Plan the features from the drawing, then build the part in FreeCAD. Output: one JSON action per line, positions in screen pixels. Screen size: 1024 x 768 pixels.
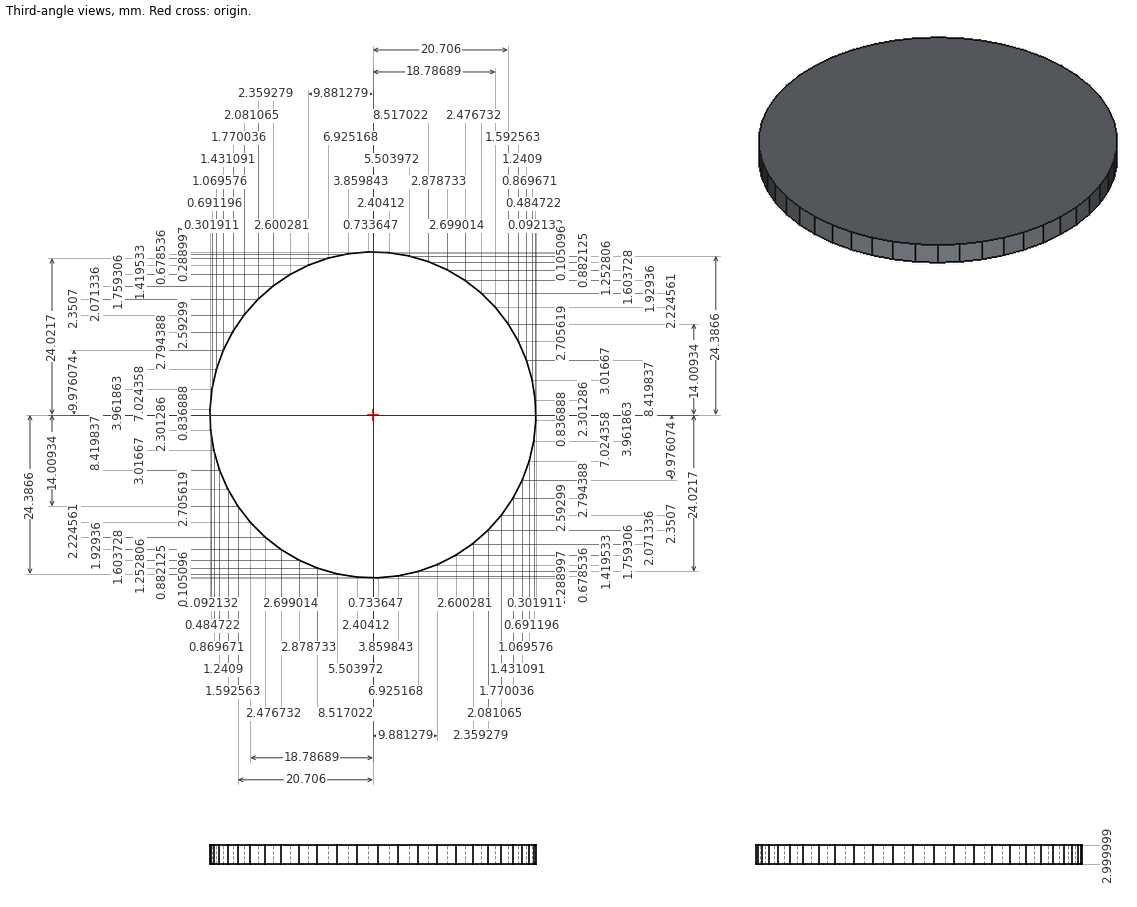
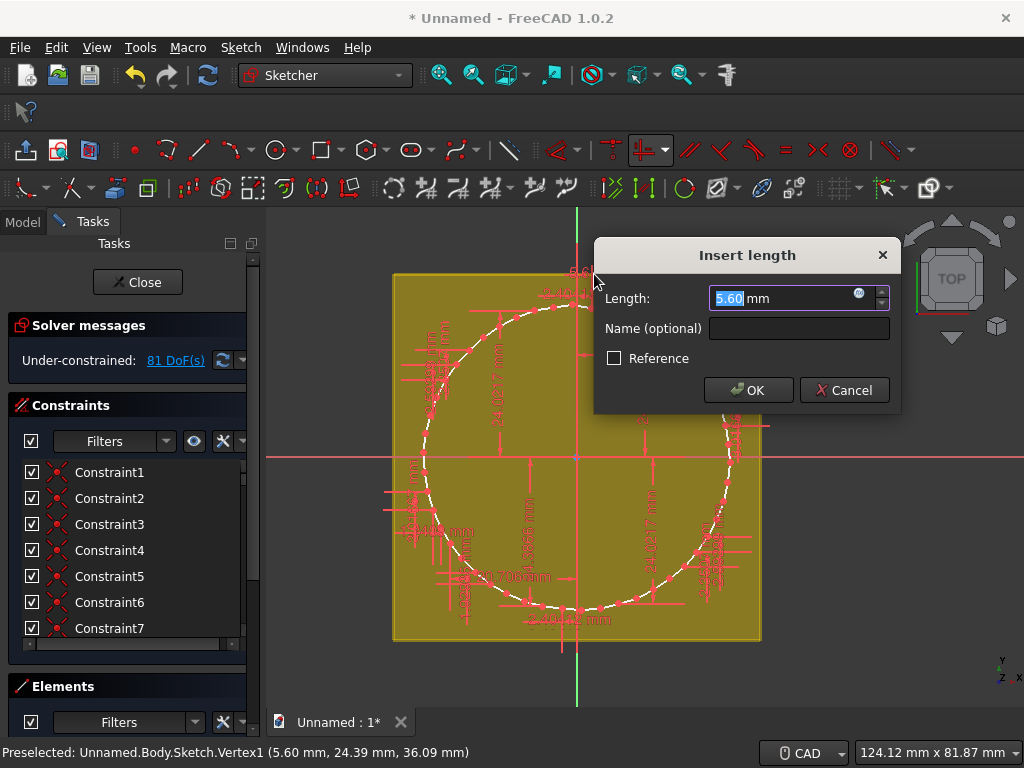
{"action": "type", "text": "5.503972"}
{"action": "key", "text": "Return"}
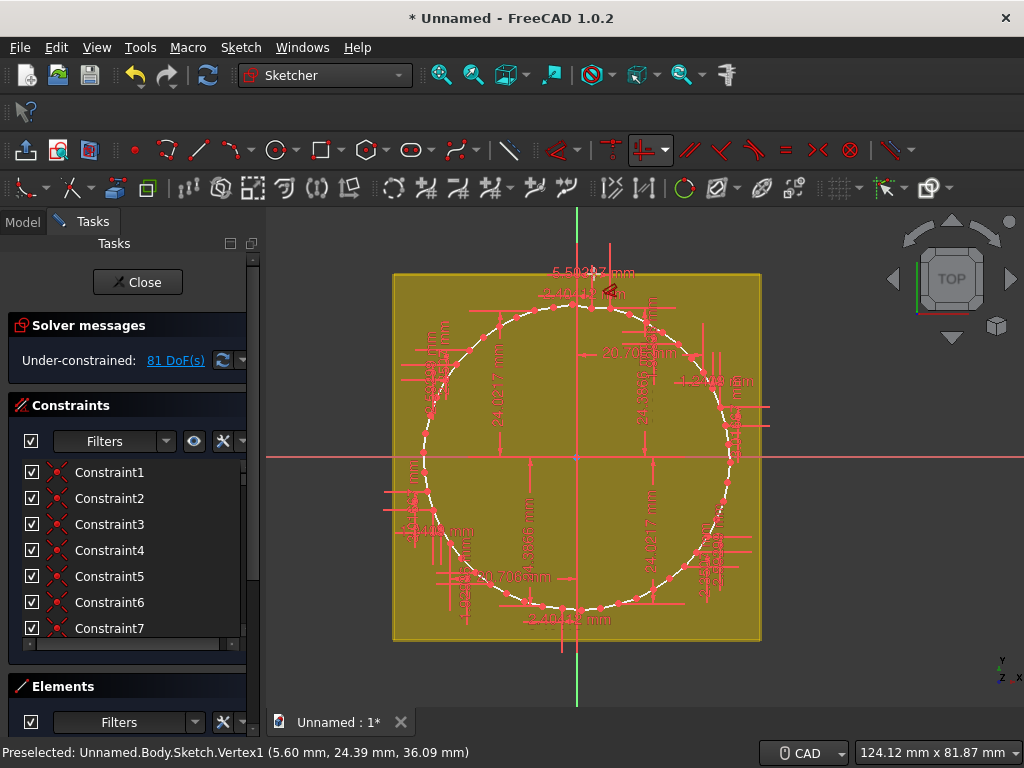
{"action": "left_click", "coordinate": [629, 314]}
{"action": "left_click", "coordinate": [603, 491]}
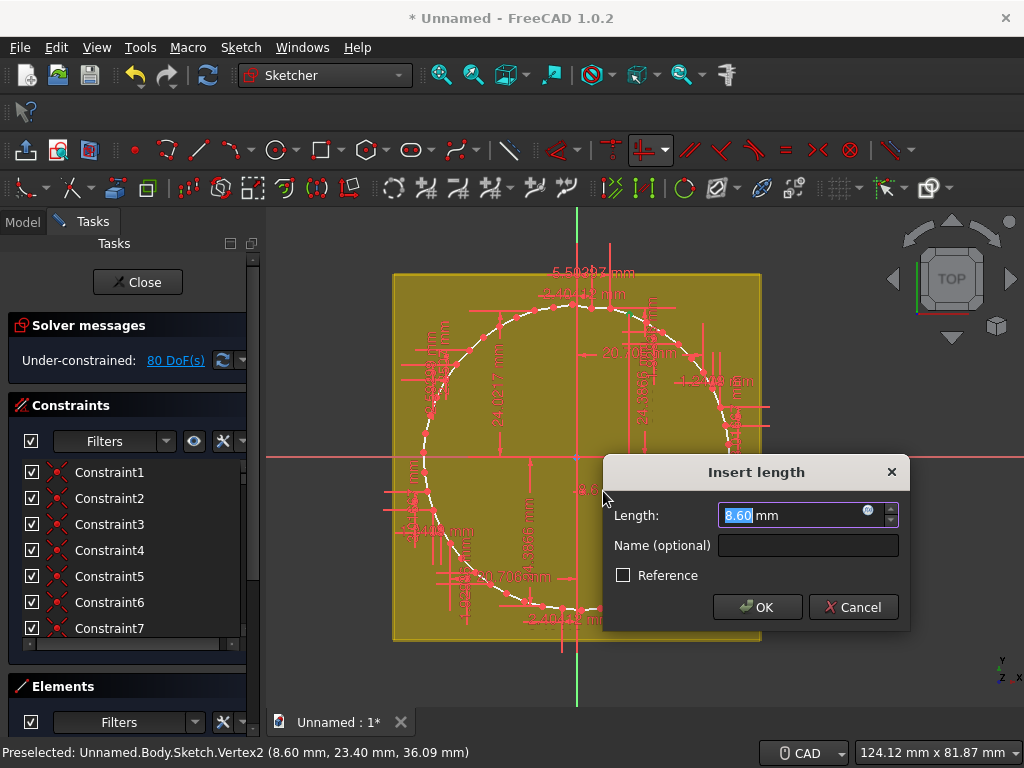
{"action": "type", "text": "8.517022"}
{"action": "key", "text": "Return"}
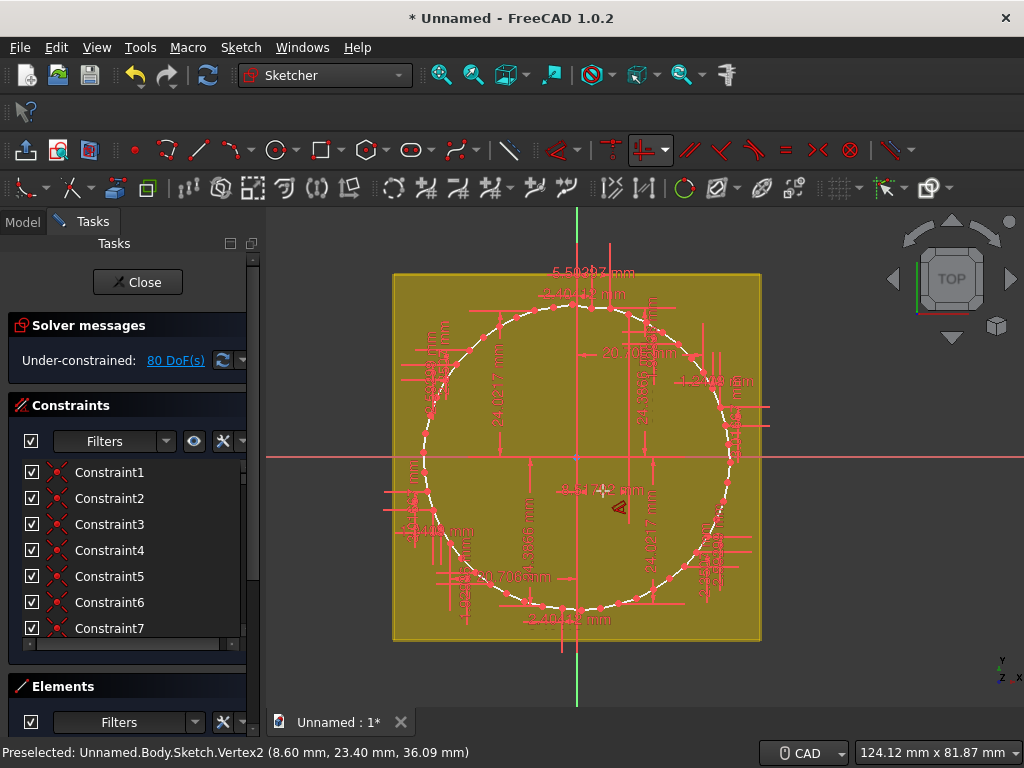
{"action": "left_click", "coordinate": [692, 358]}
{"action": "left_click", "coordinate": [674, 491]}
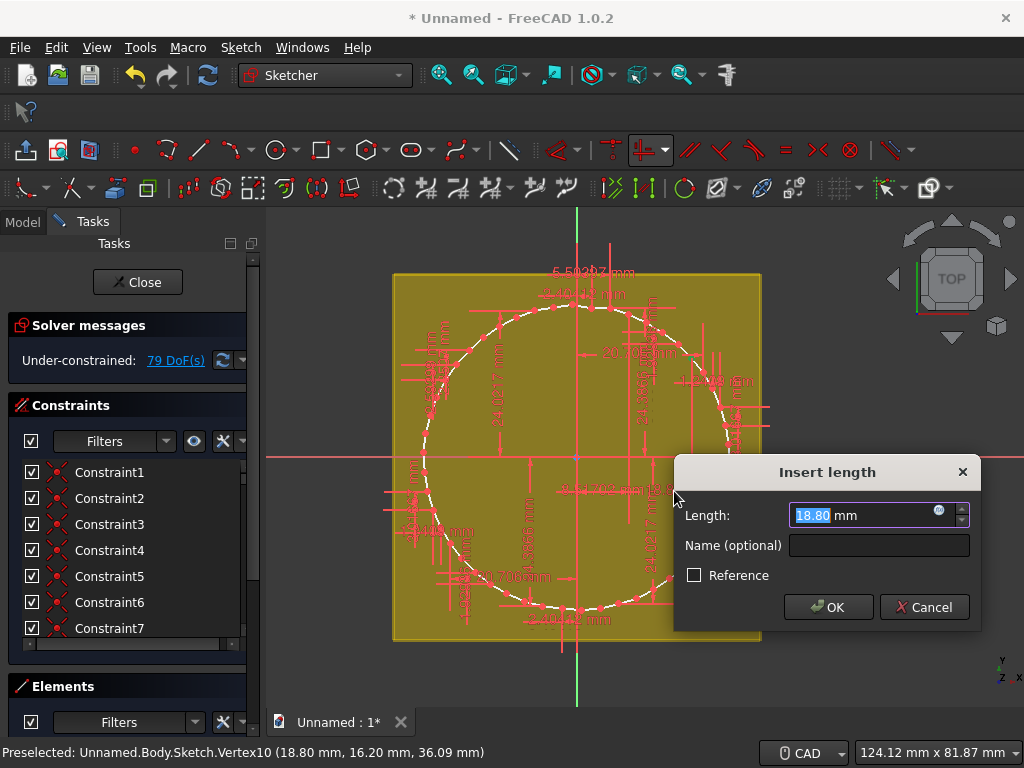
{"action": "type", "text": "18.78689"}
{"action": "key", "text": "Return"}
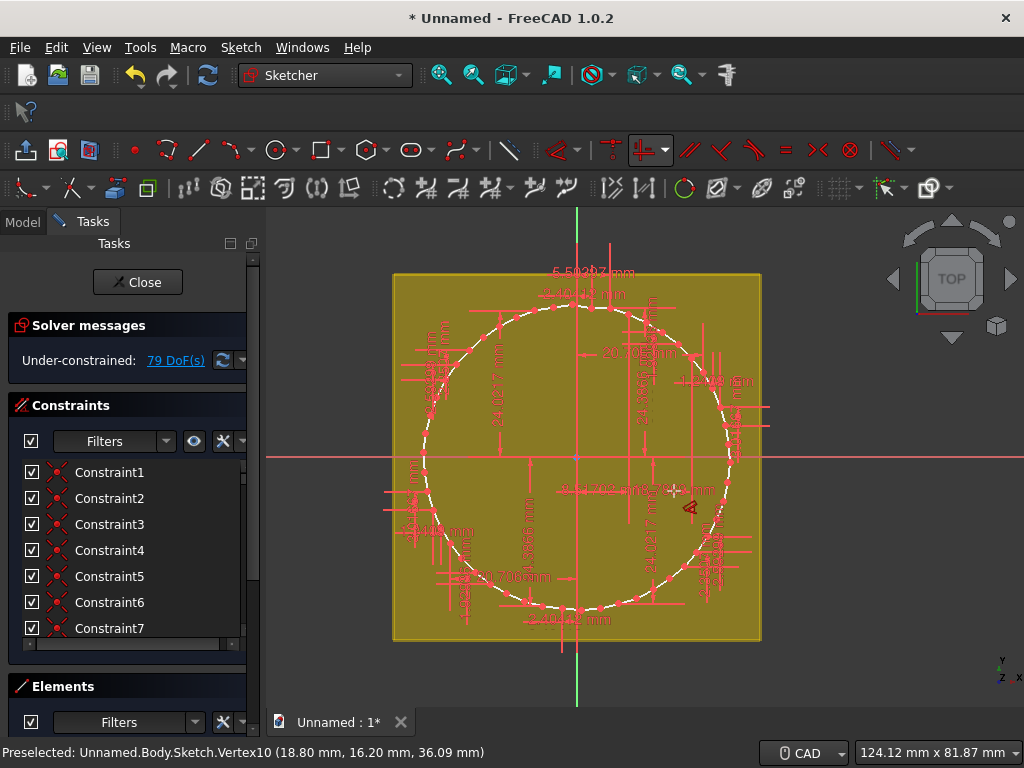
{"action": "left_click", "coordinate": [703, 373]}
{"action": "left_click", "coordinate": [543, 415]}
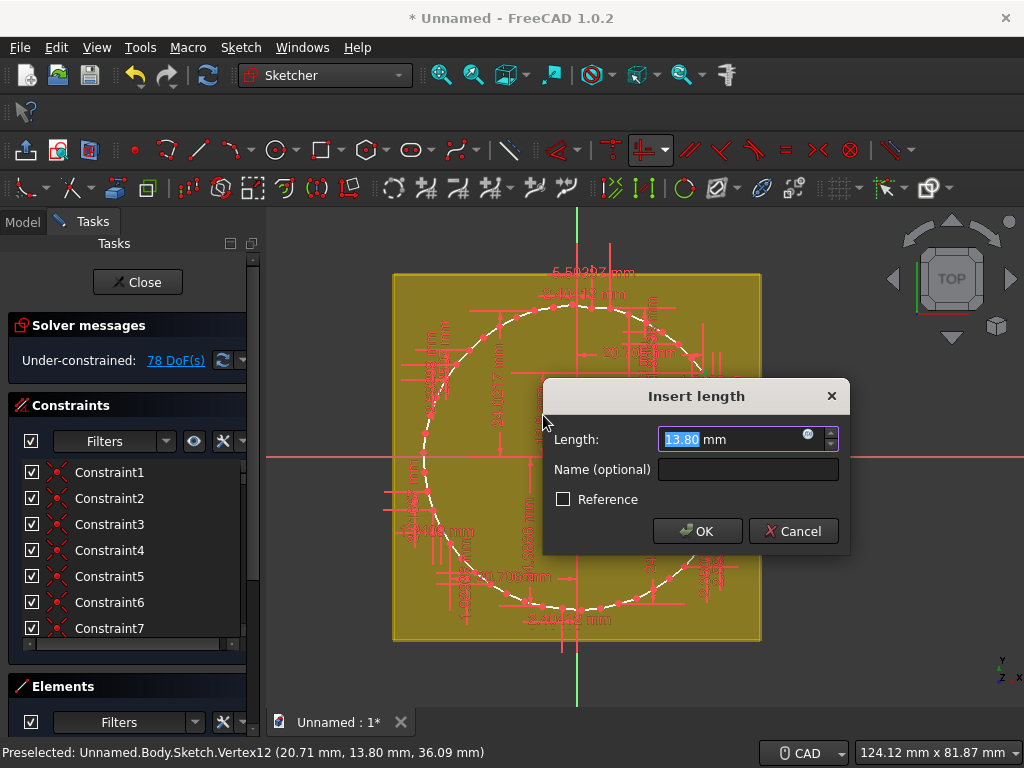
{"action": "type", "text": "14.00934"}
{"action": "key", "text": "Return"}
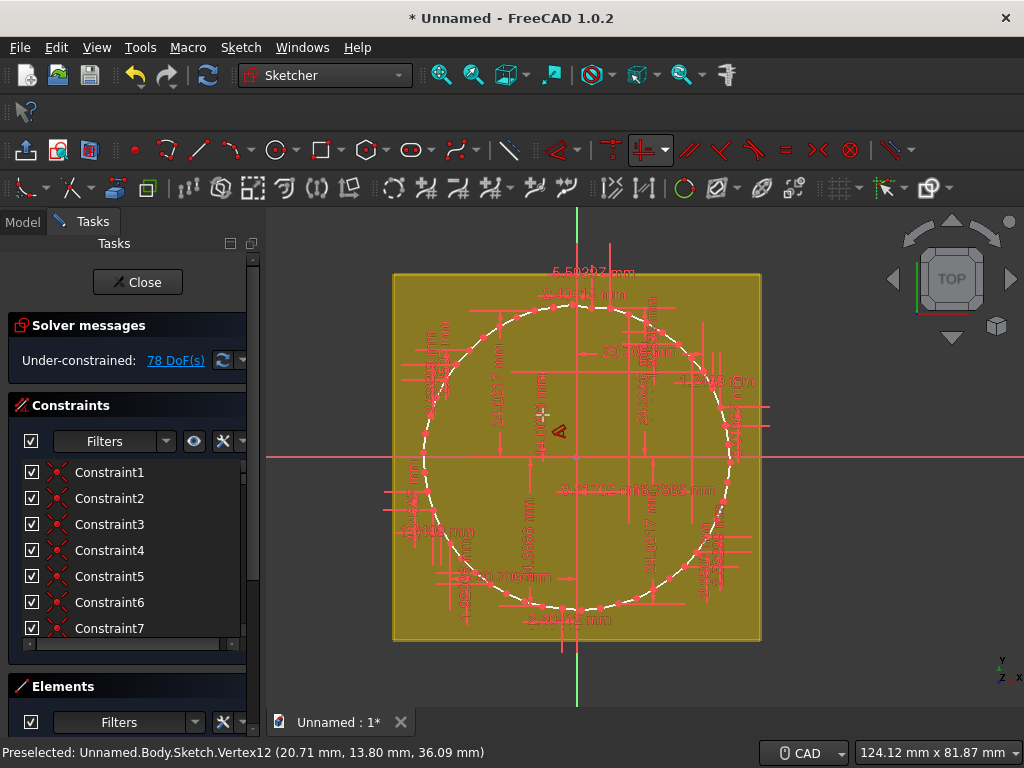
{"action": "left_click", "coordinate": [720, 407]}
{"action": "left_click", "coordinate": [754, 444]}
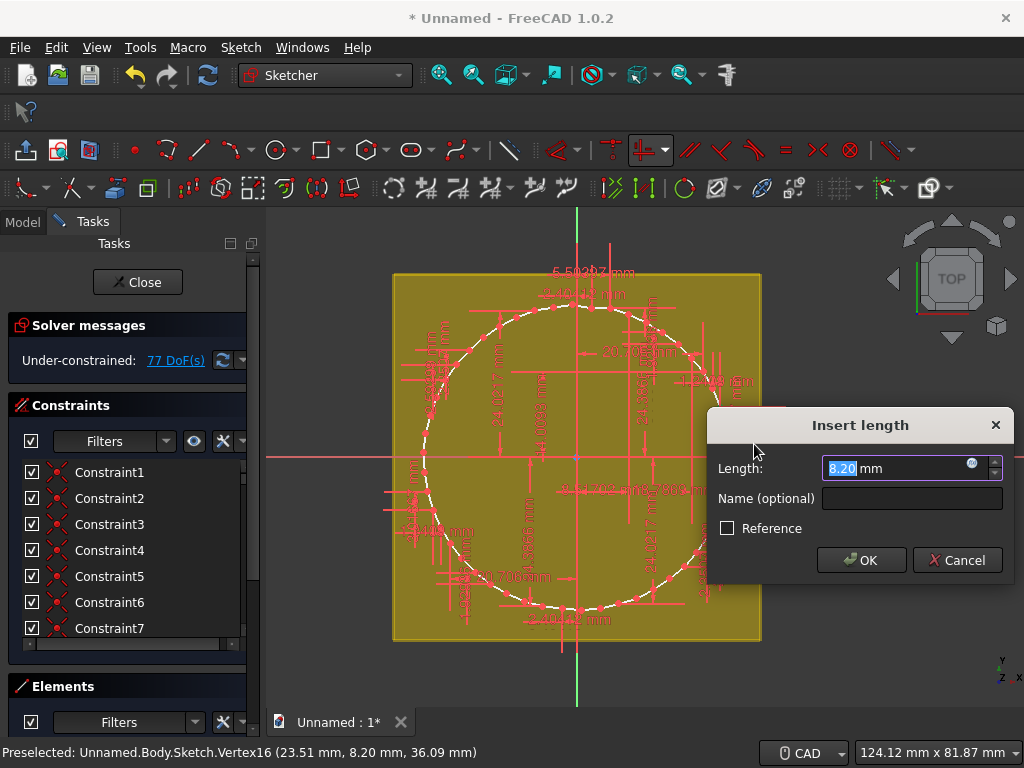
{"action": "type", "text": "8.419837"}
{"action": "key", "text": "Return"}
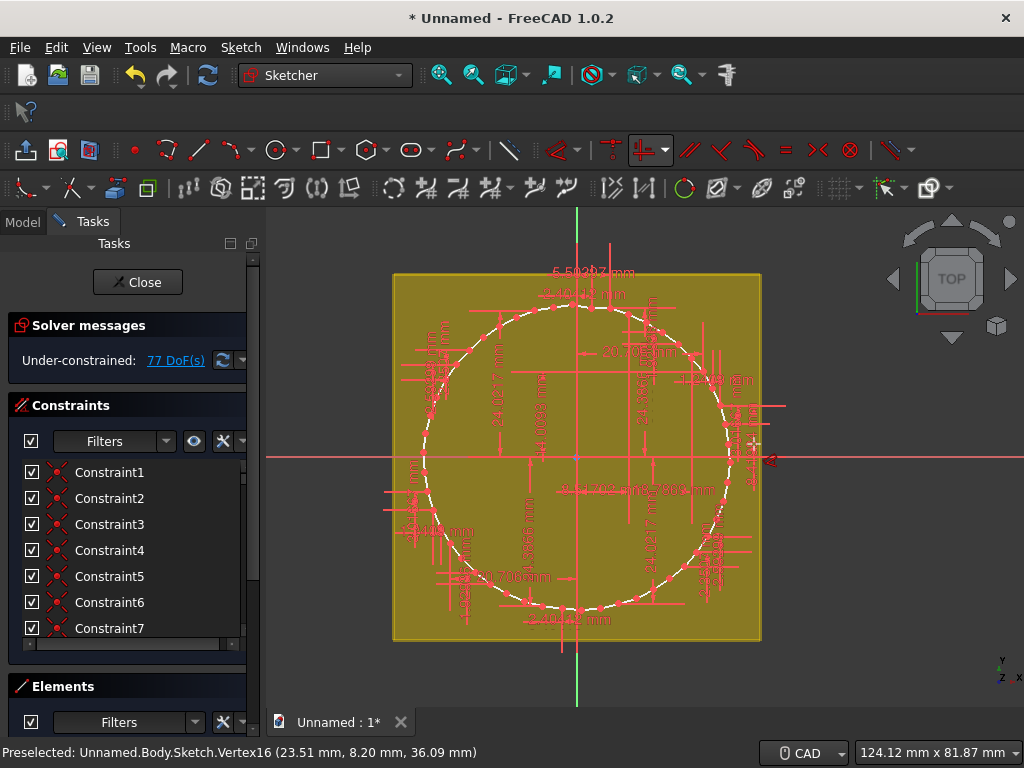
{"action": "scroll", "coordinate": [729, 444], "scroll_direction": "up", "scroll_amount": 6}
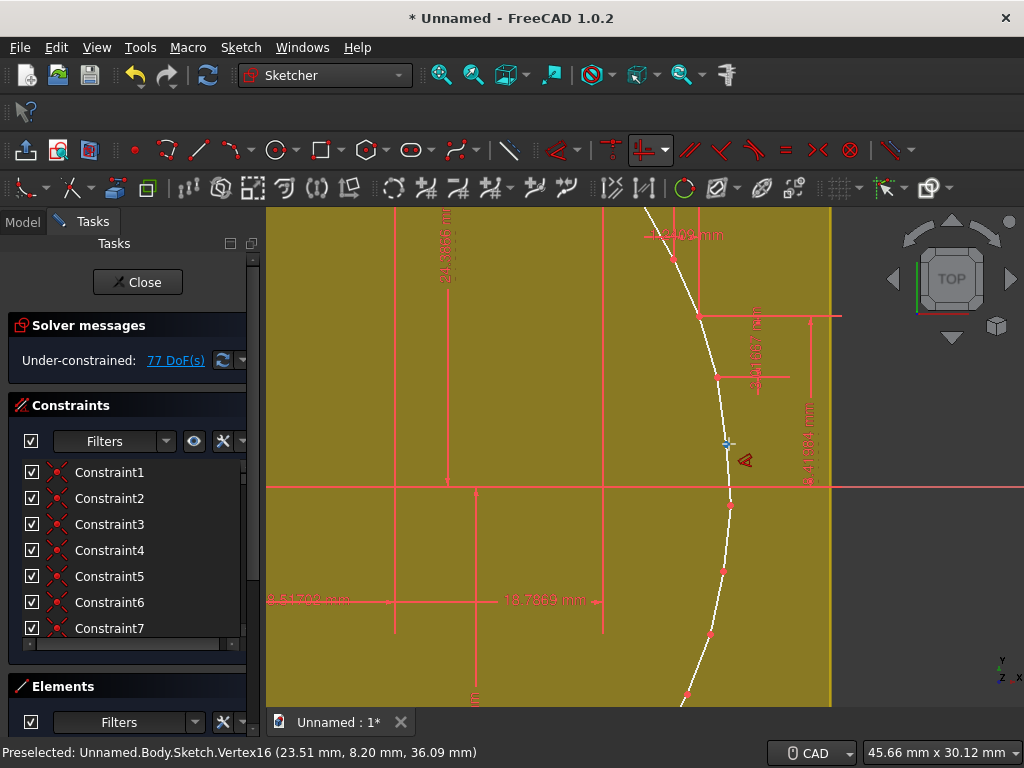
{"action": "left_click", "coordinate": [726, 444]}
{"action": "left_click", "coordinate": [760, 466]}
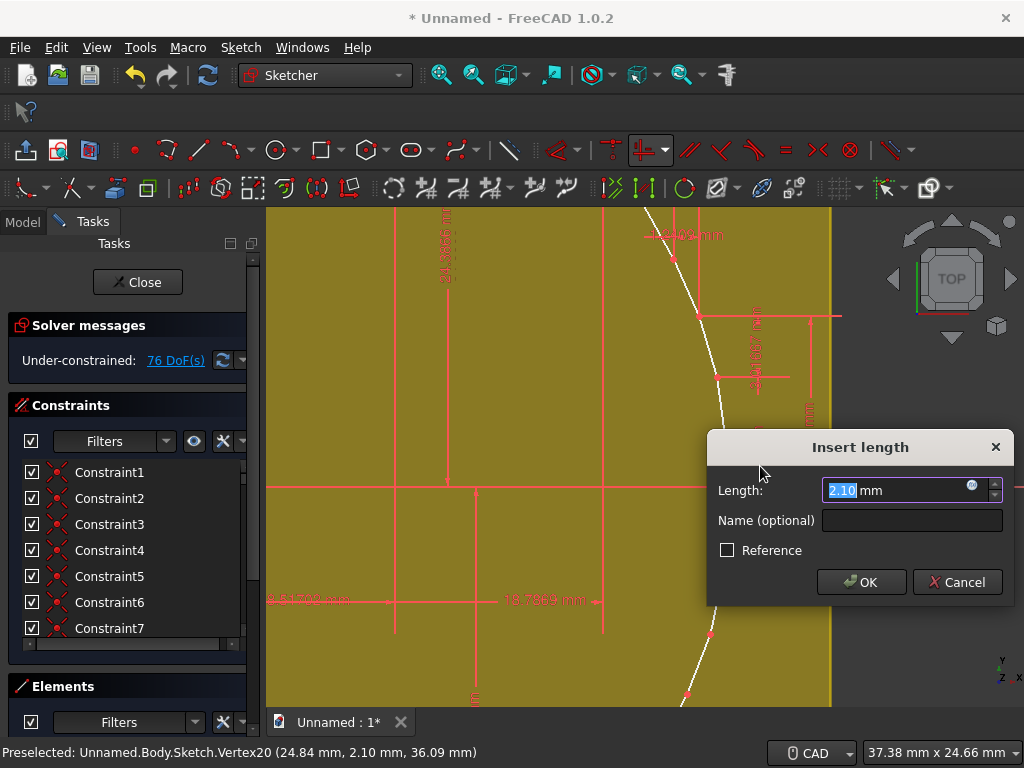
{"action": "type", "text": "2.301286"}
{"action": "key", "text": "Return"}